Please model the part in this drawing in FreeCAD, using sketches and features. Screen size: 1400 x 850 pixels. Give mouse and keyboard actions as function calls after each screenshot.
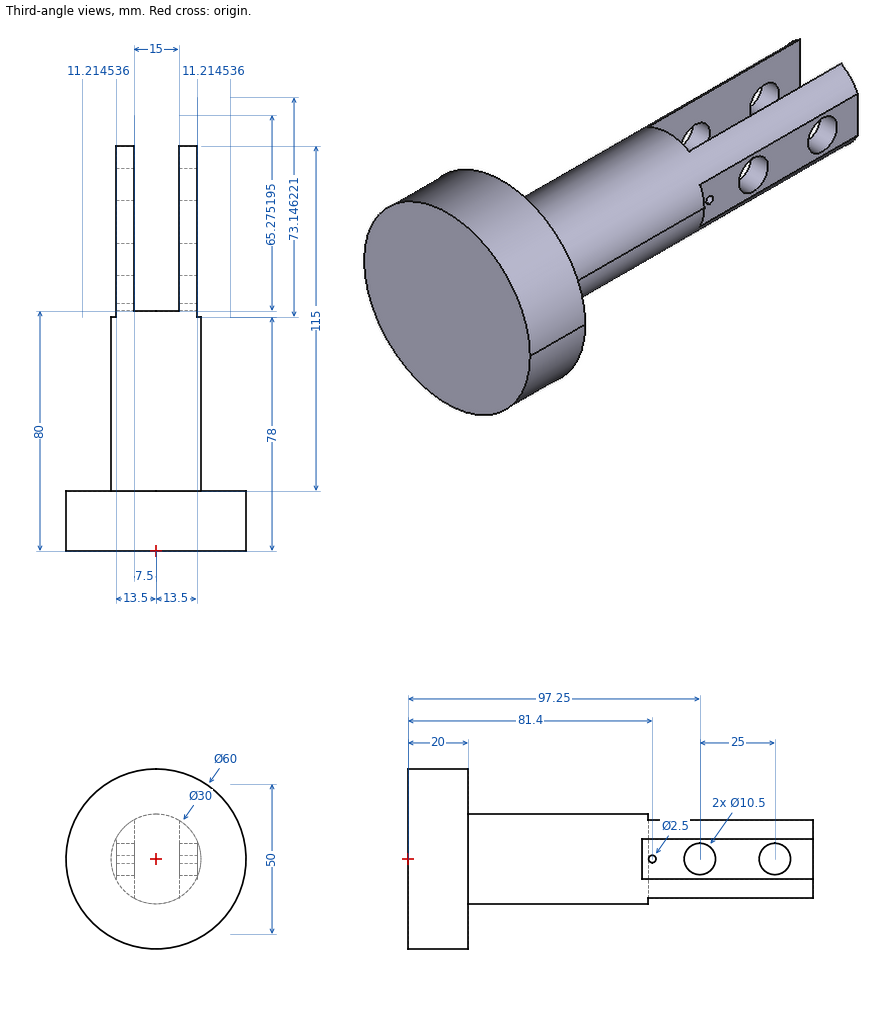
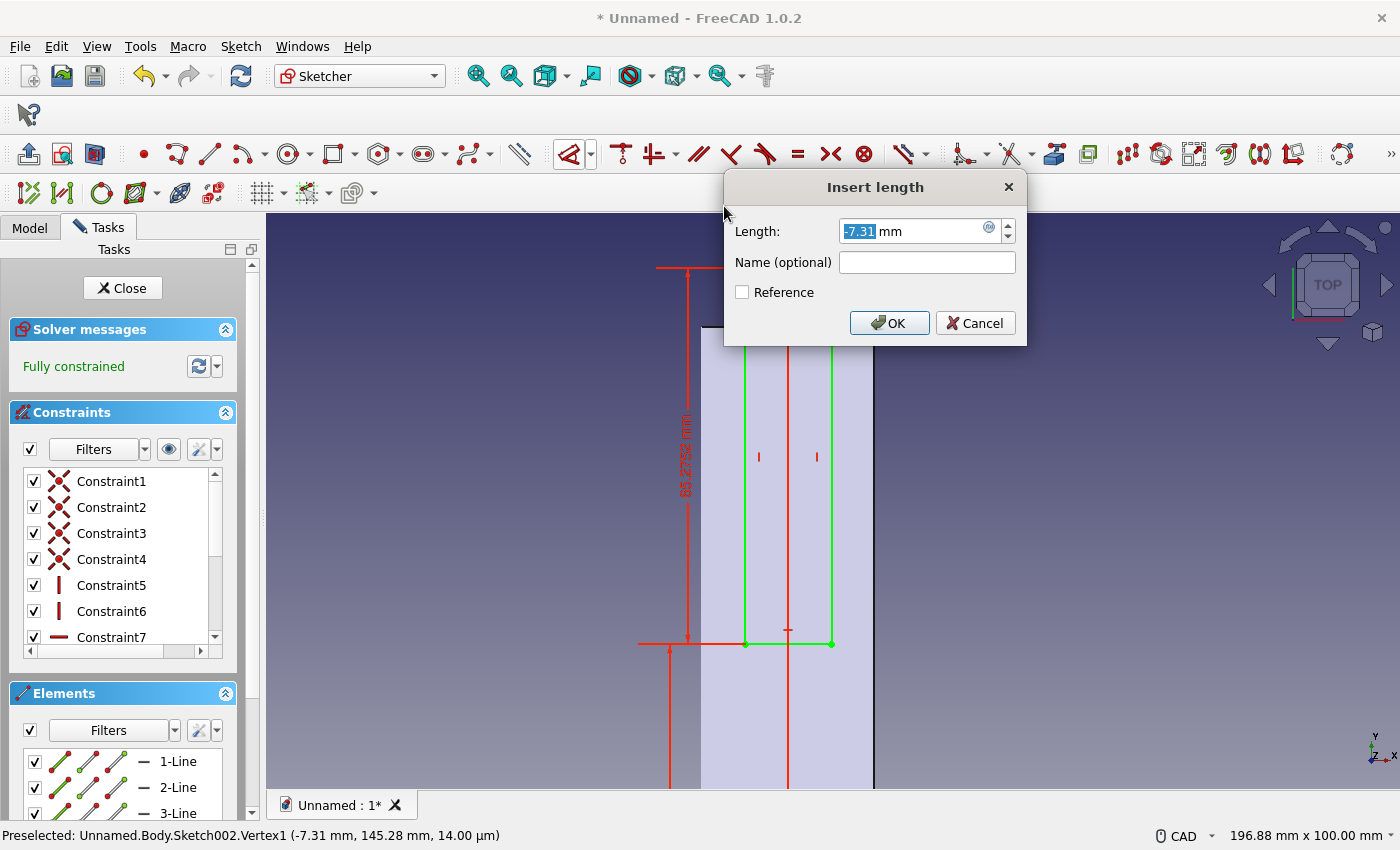
text(-7.5)
key(Return)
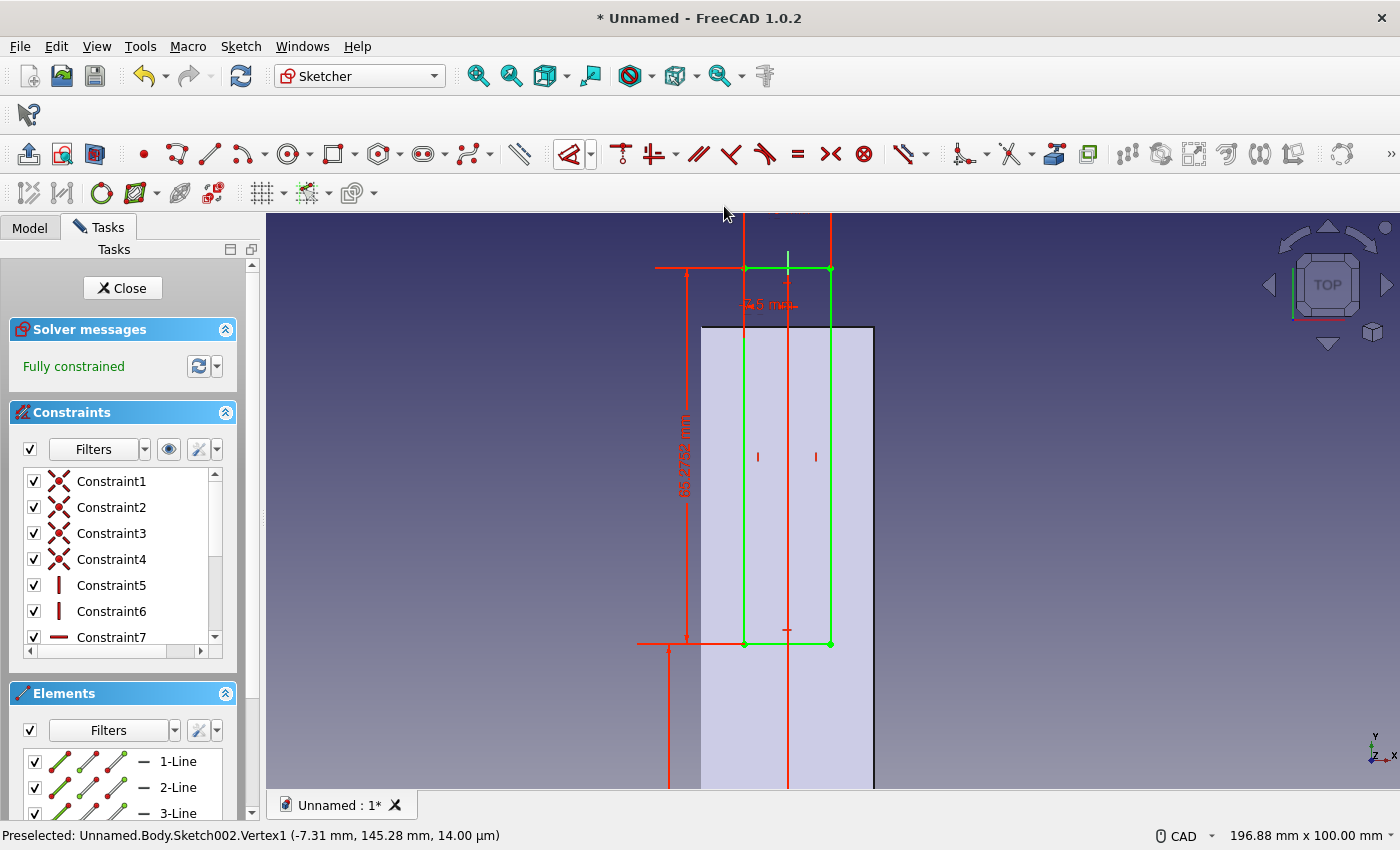
click(123, 288)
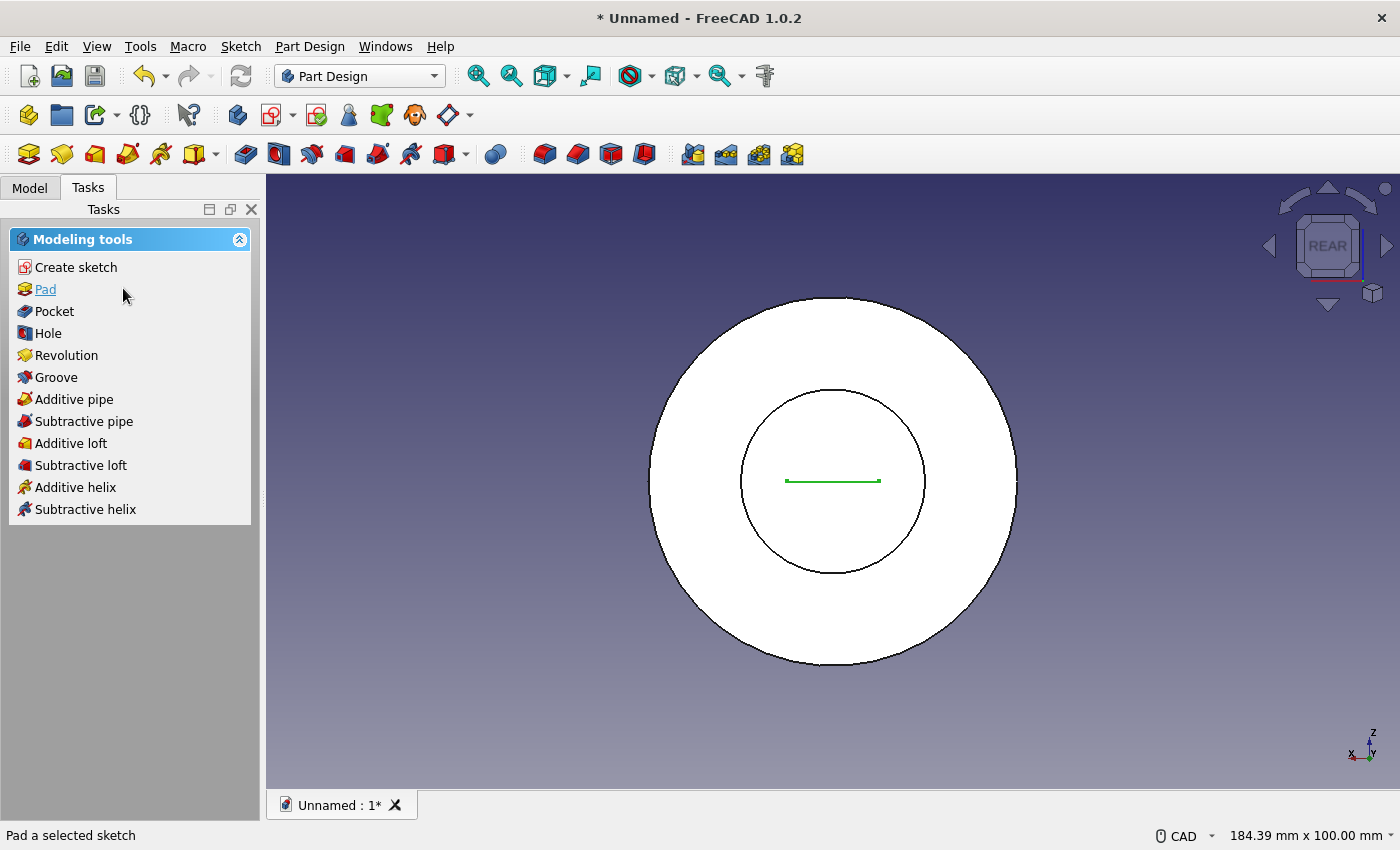
click(246, 154)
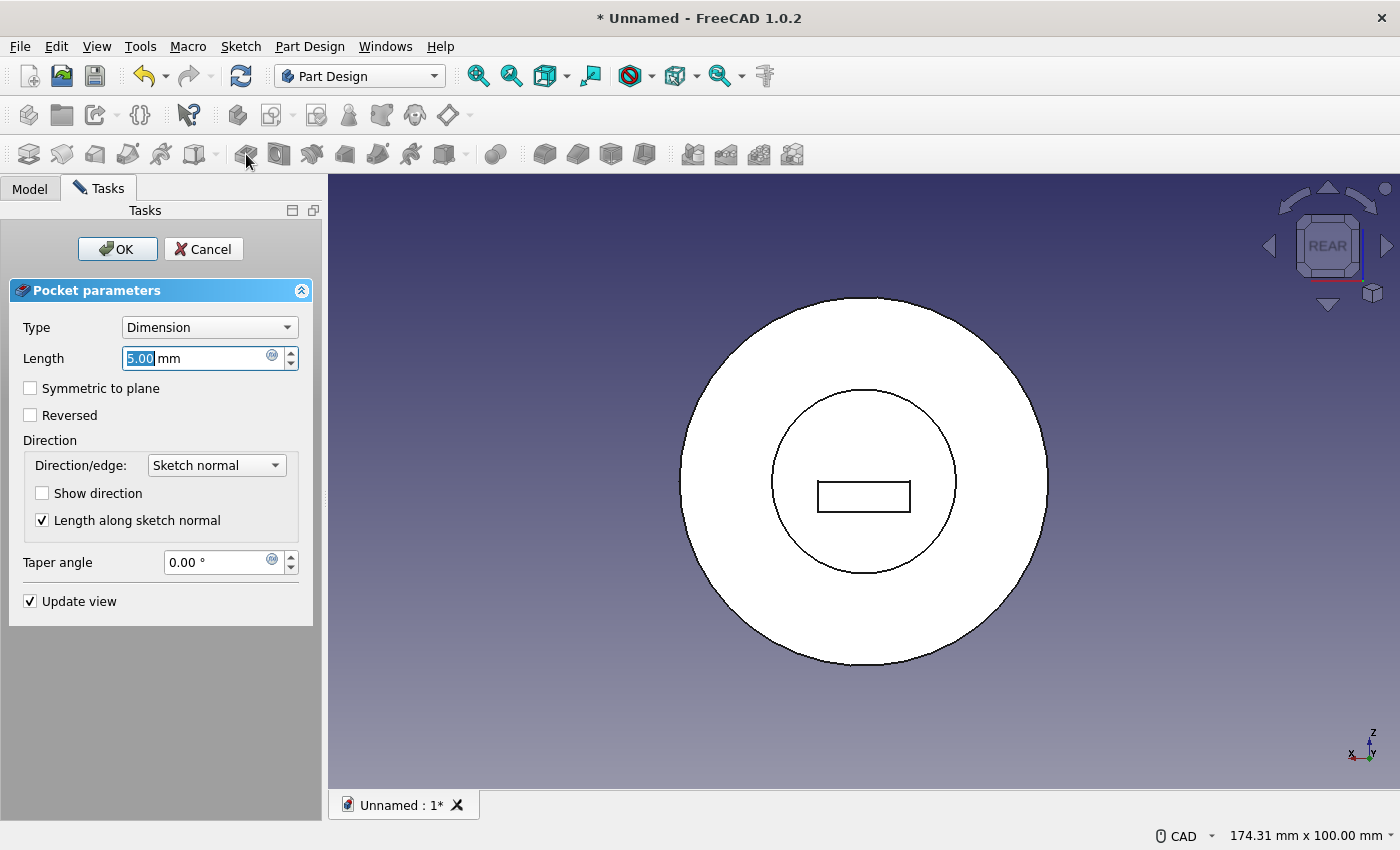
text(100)
key(Tab)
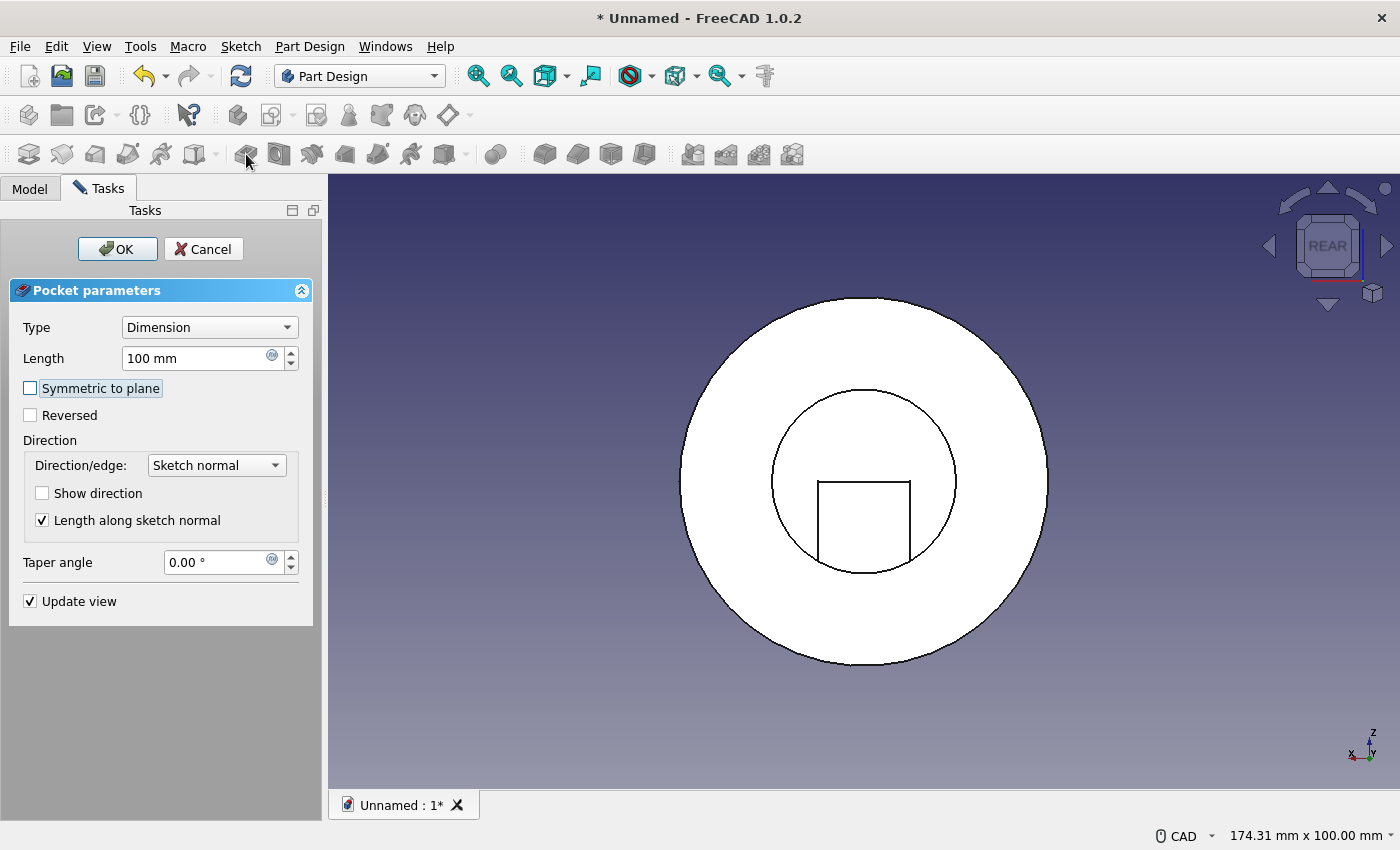
click(31, 388)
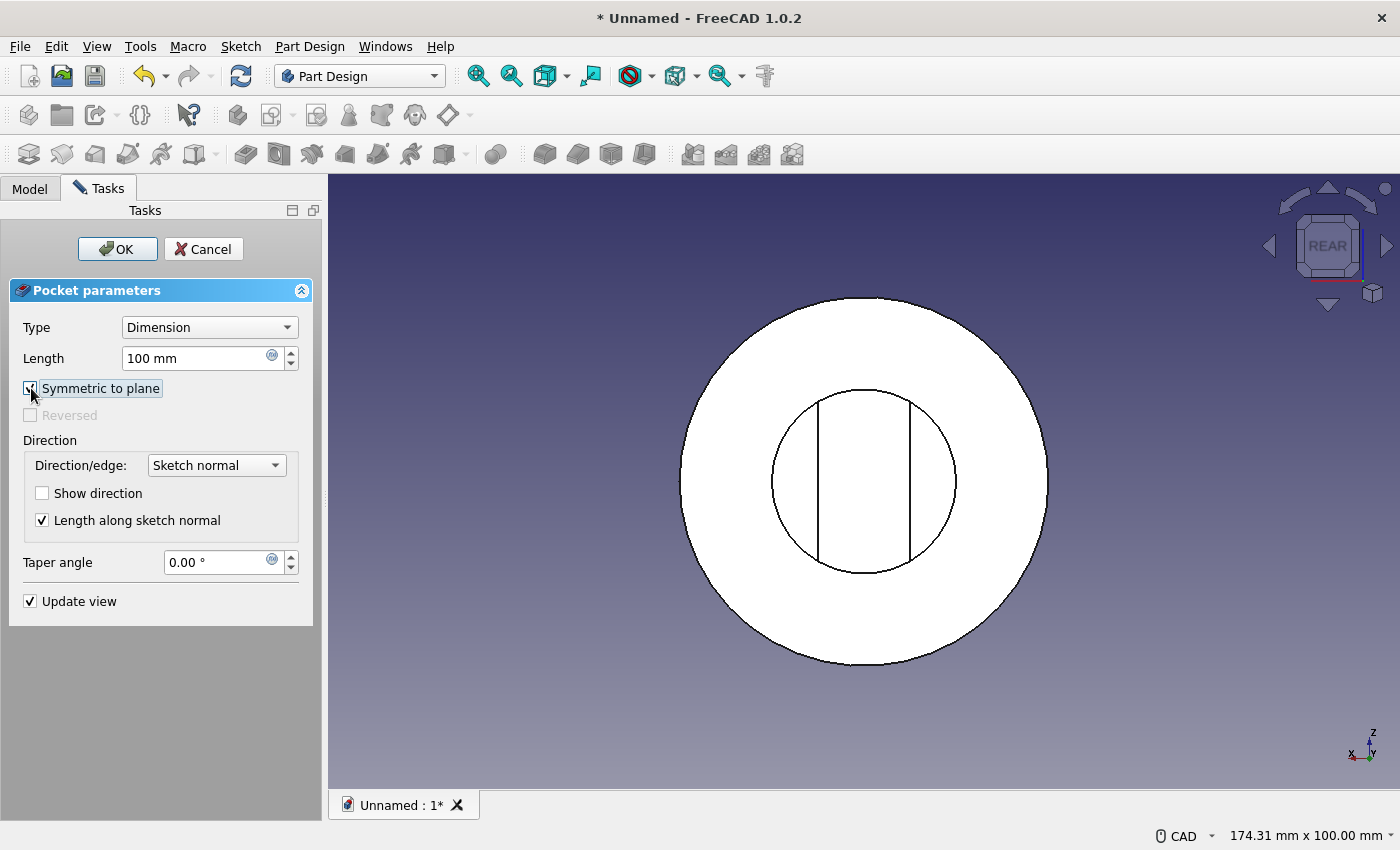
click(118, 249)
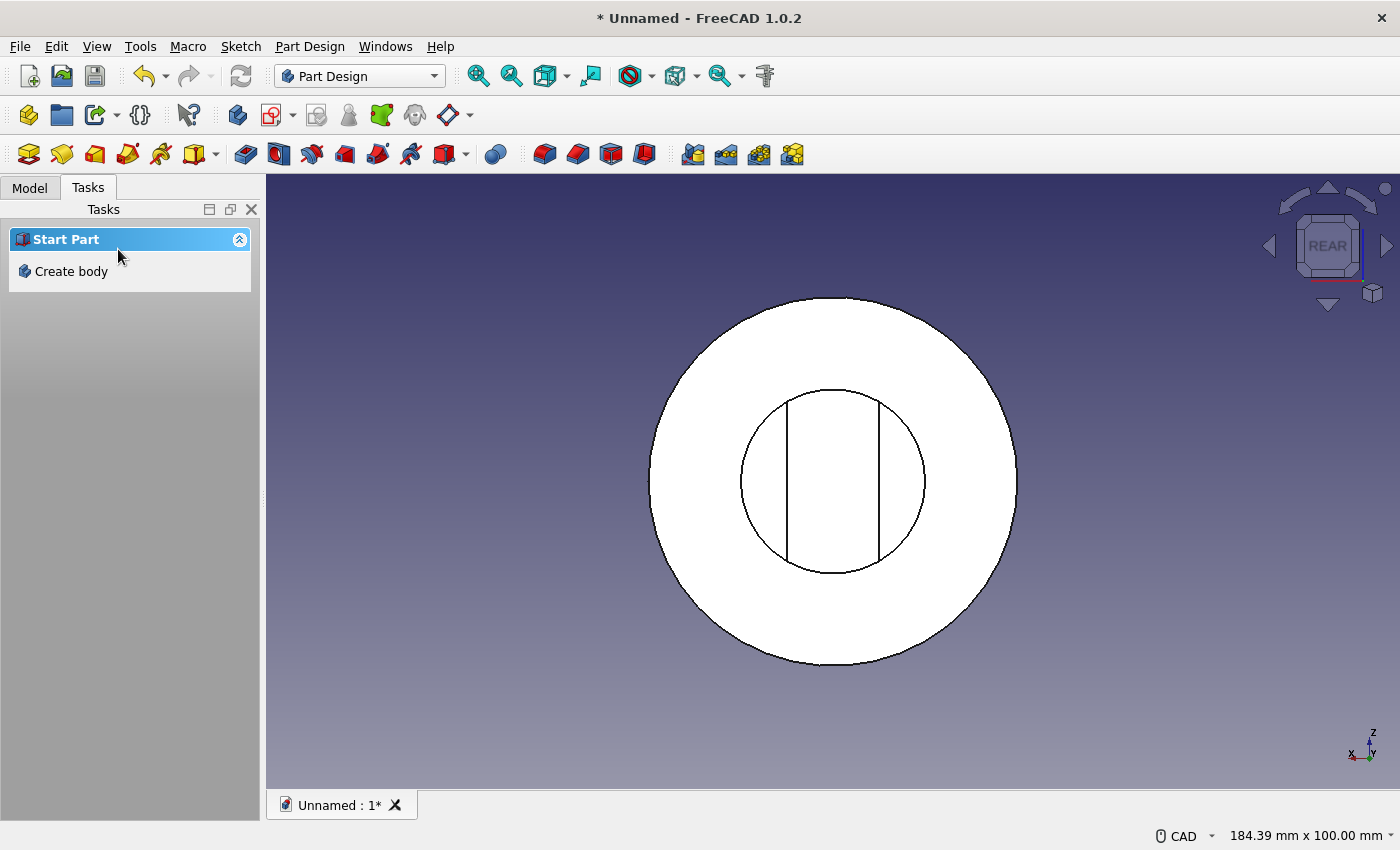
click(270, 116)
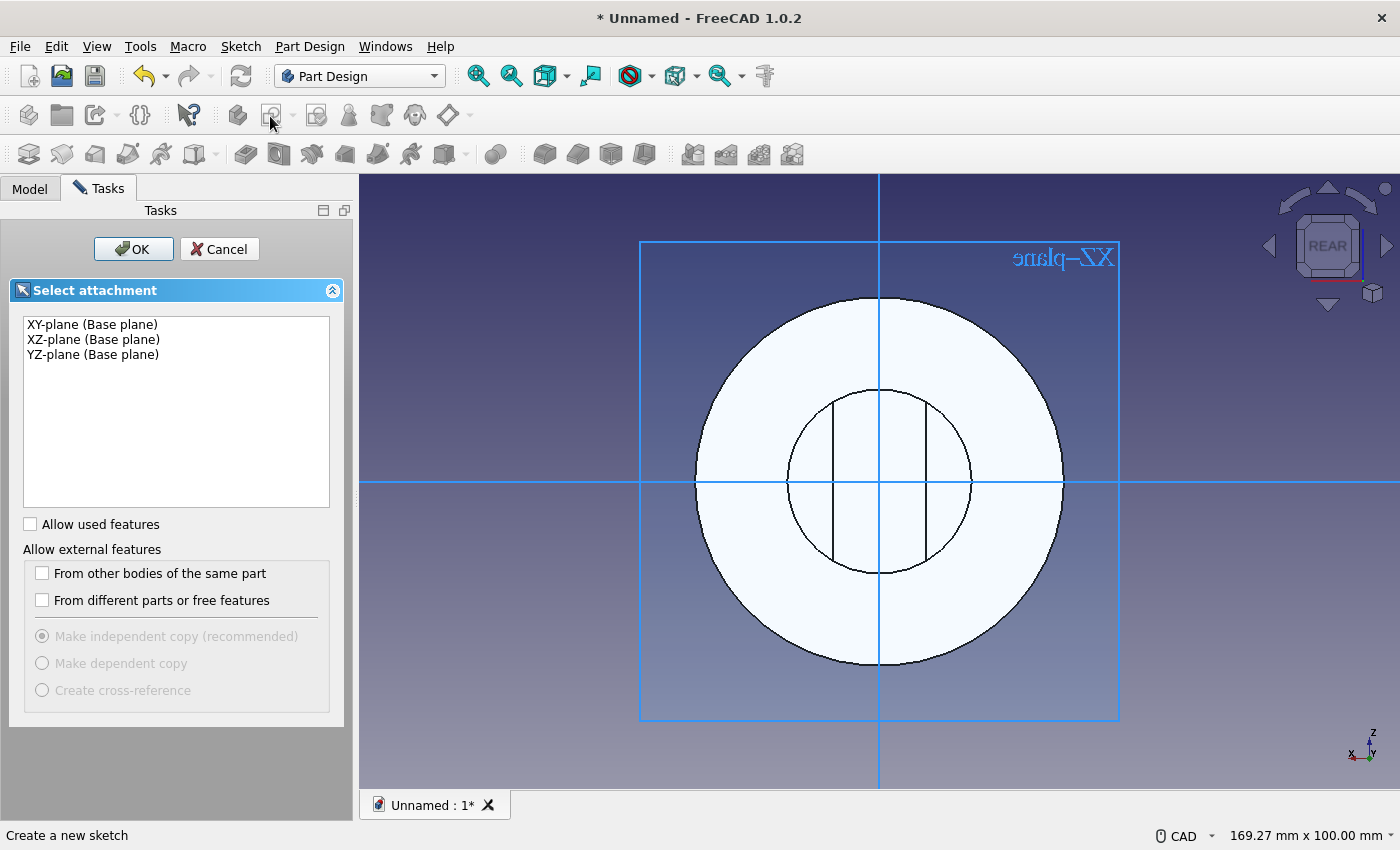
click(84, 324)